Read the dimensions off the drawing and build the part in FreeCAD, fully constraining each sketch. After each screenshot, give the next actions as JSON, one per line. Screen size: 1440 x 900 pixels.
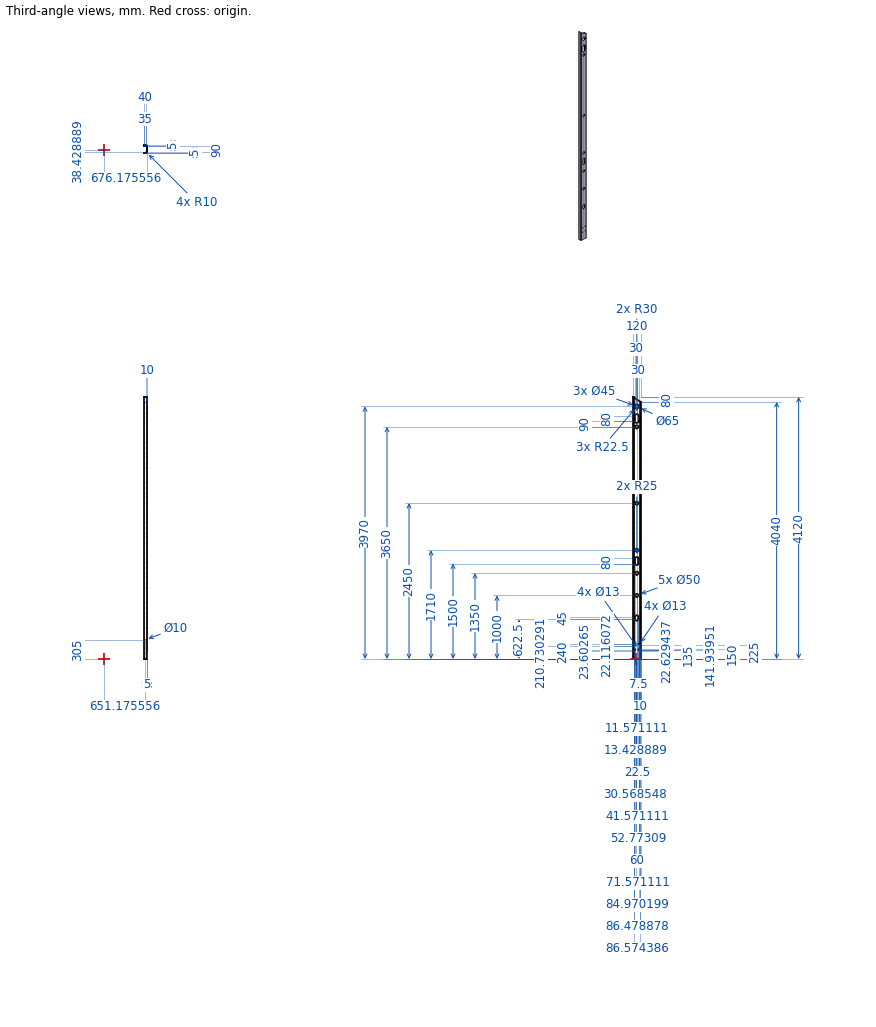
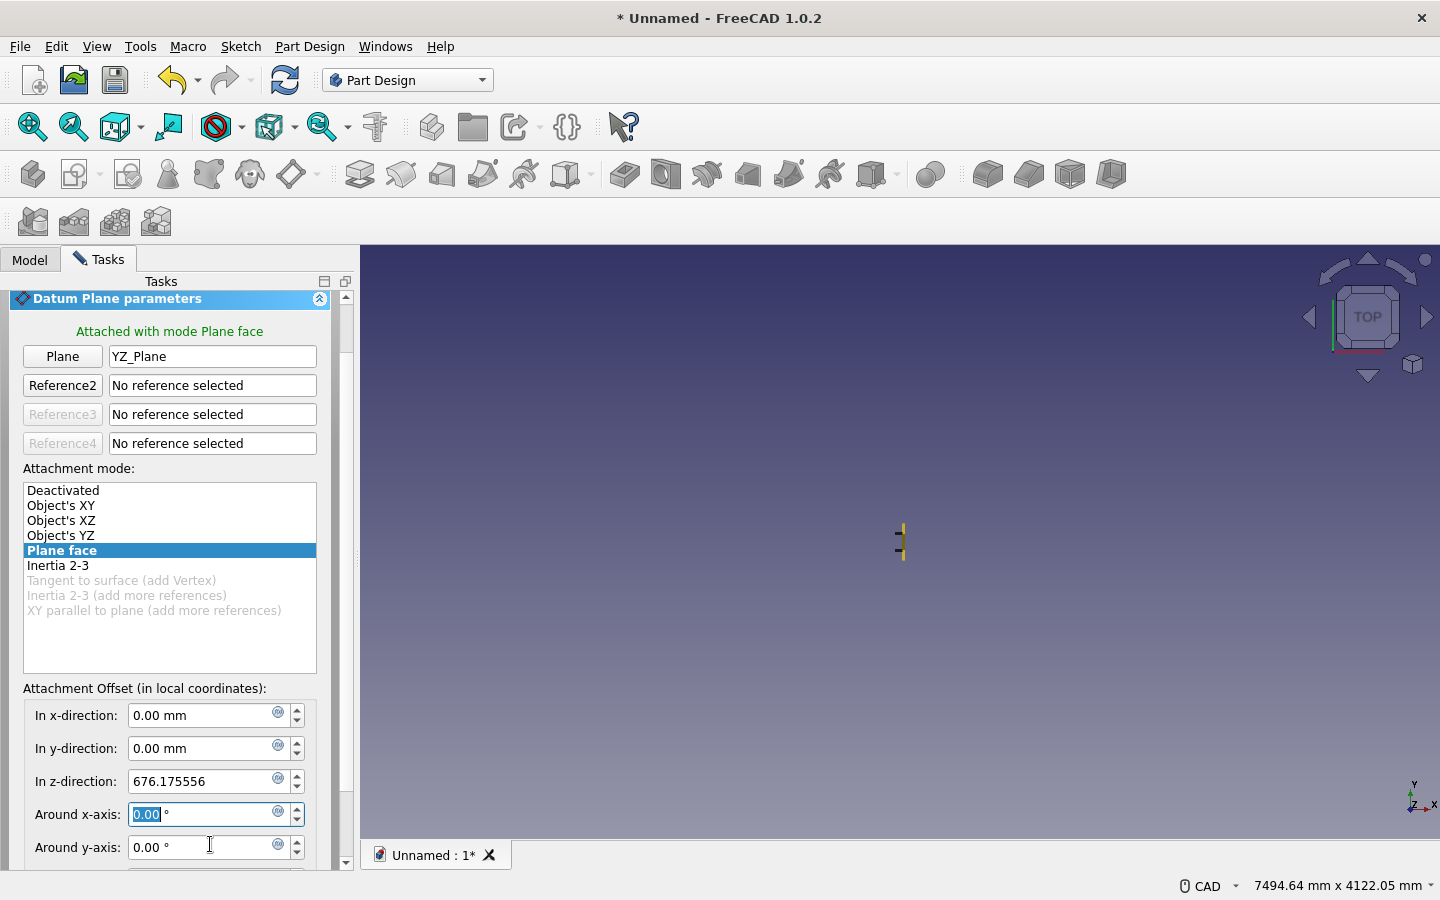
{"action": "scroll", "coordinate": [346, 580], "scroll_direction": "up", "scroll_amount": 2}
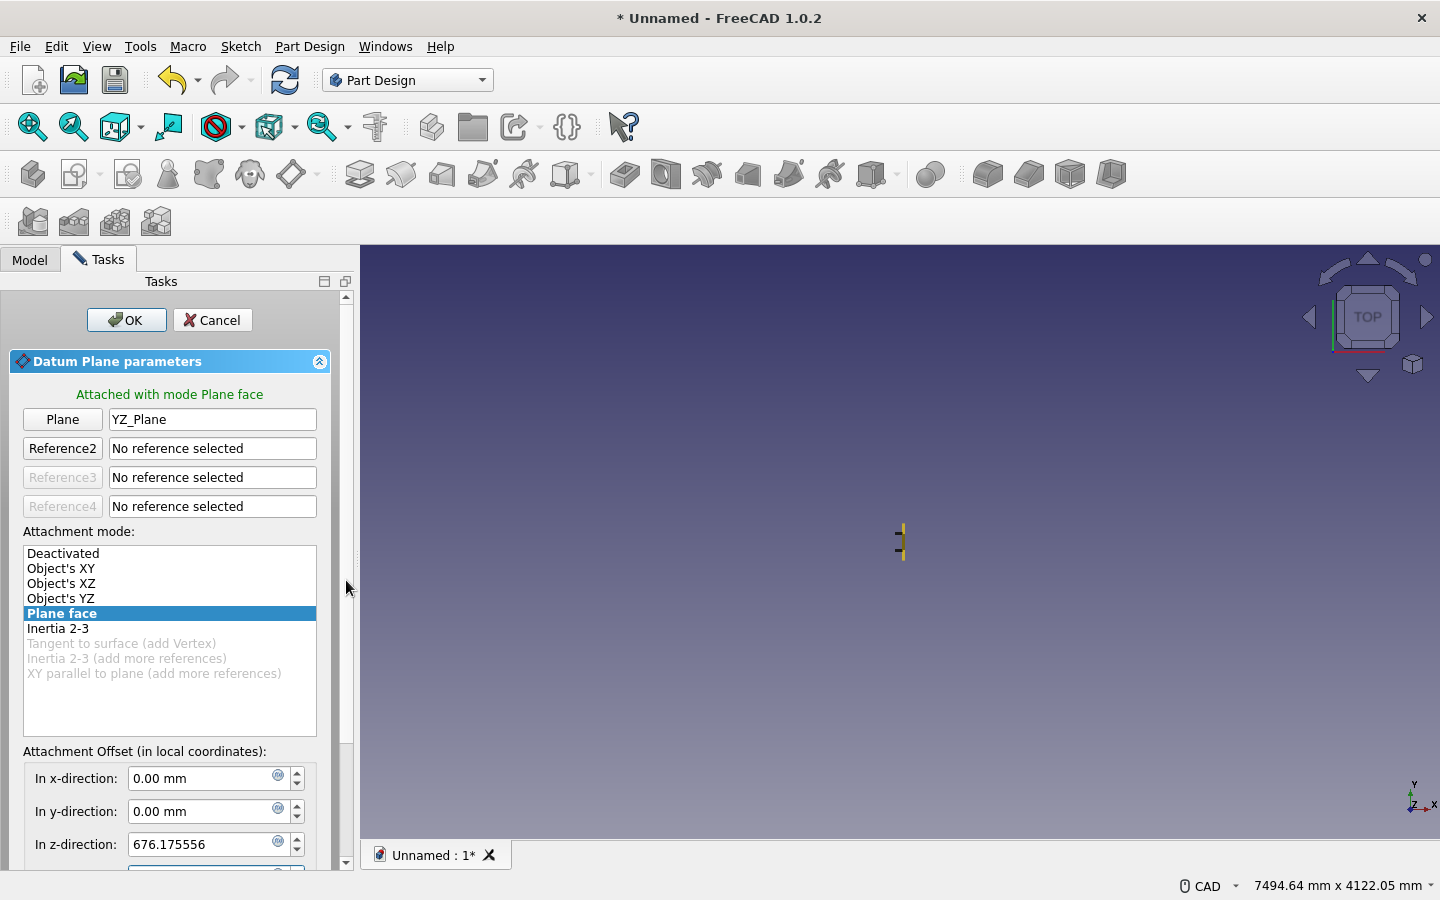
{"action": "left_click", "coordinate": [127, 320]}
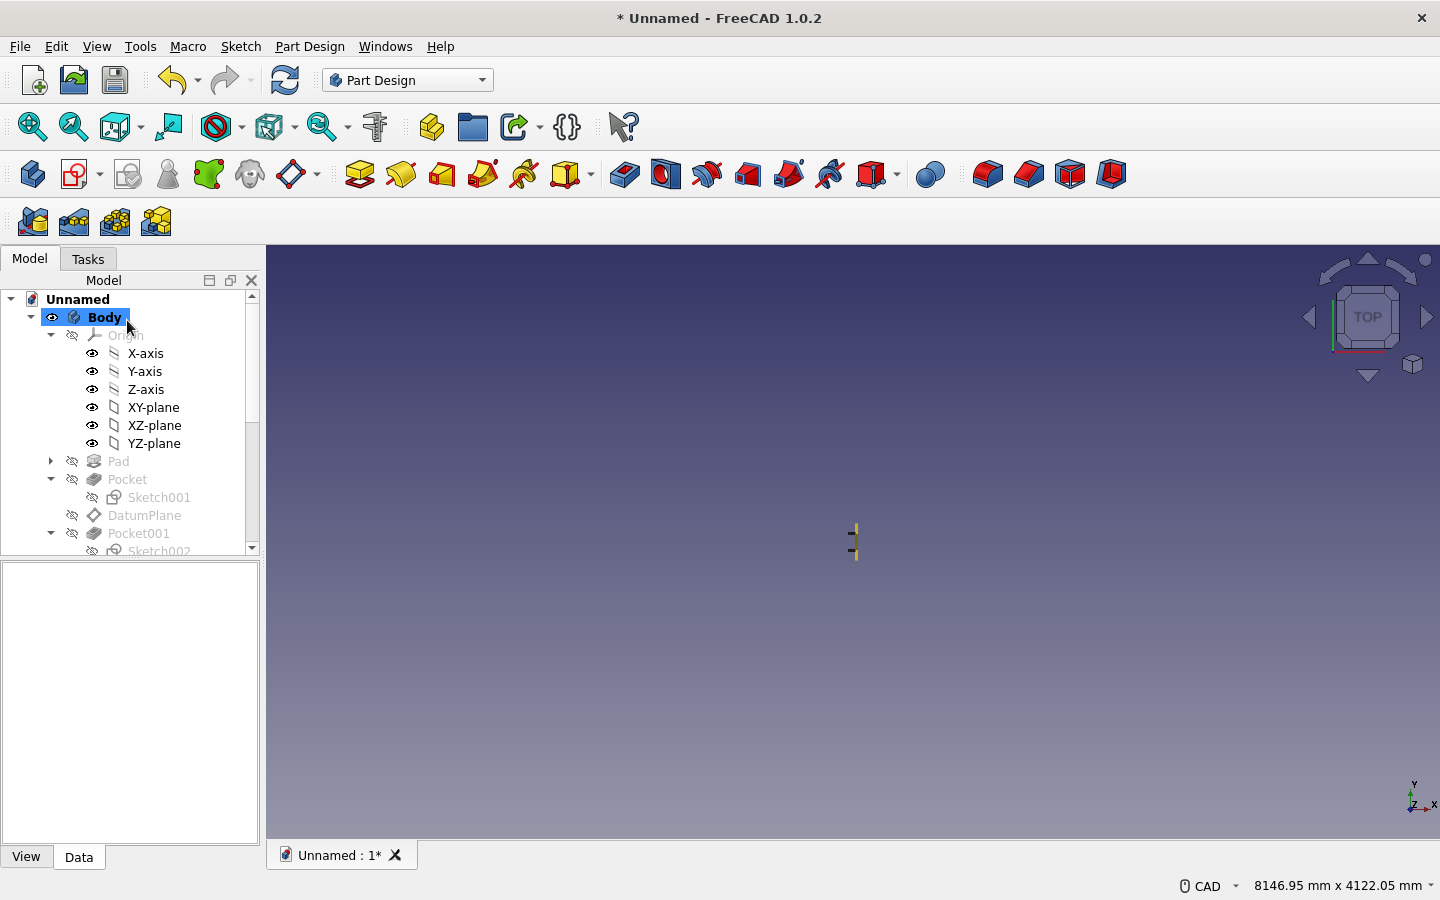
{"action": "scroll", "coordinate": [101, 421], "scroll_direction": "down", "scroll_amount": 3}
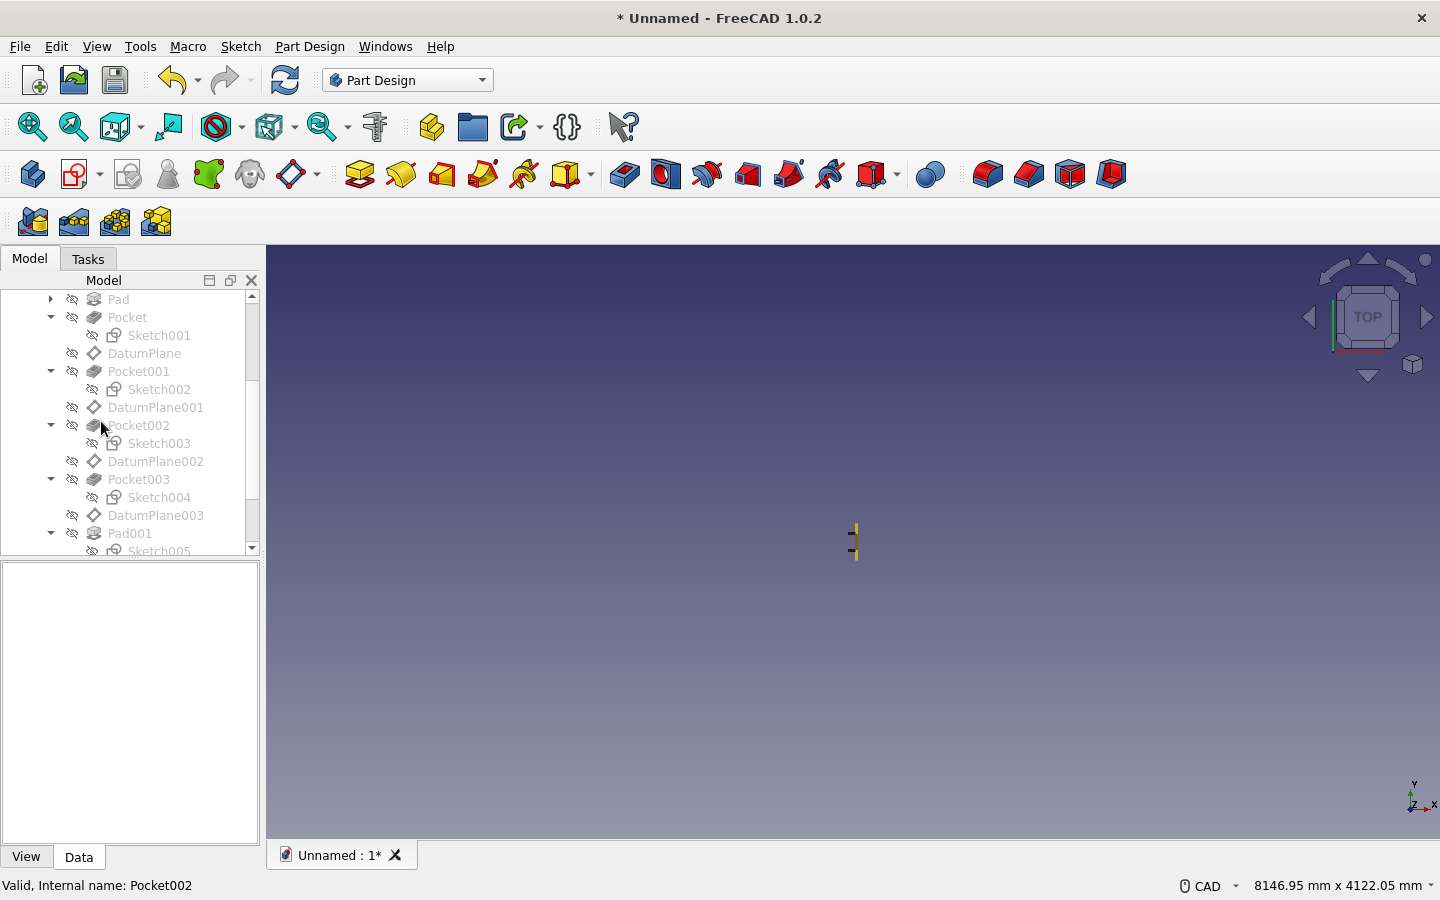
{"action": "scroll", "coordinate": [141, 421], "scroll_direction": "up", "scroll_amount": 15}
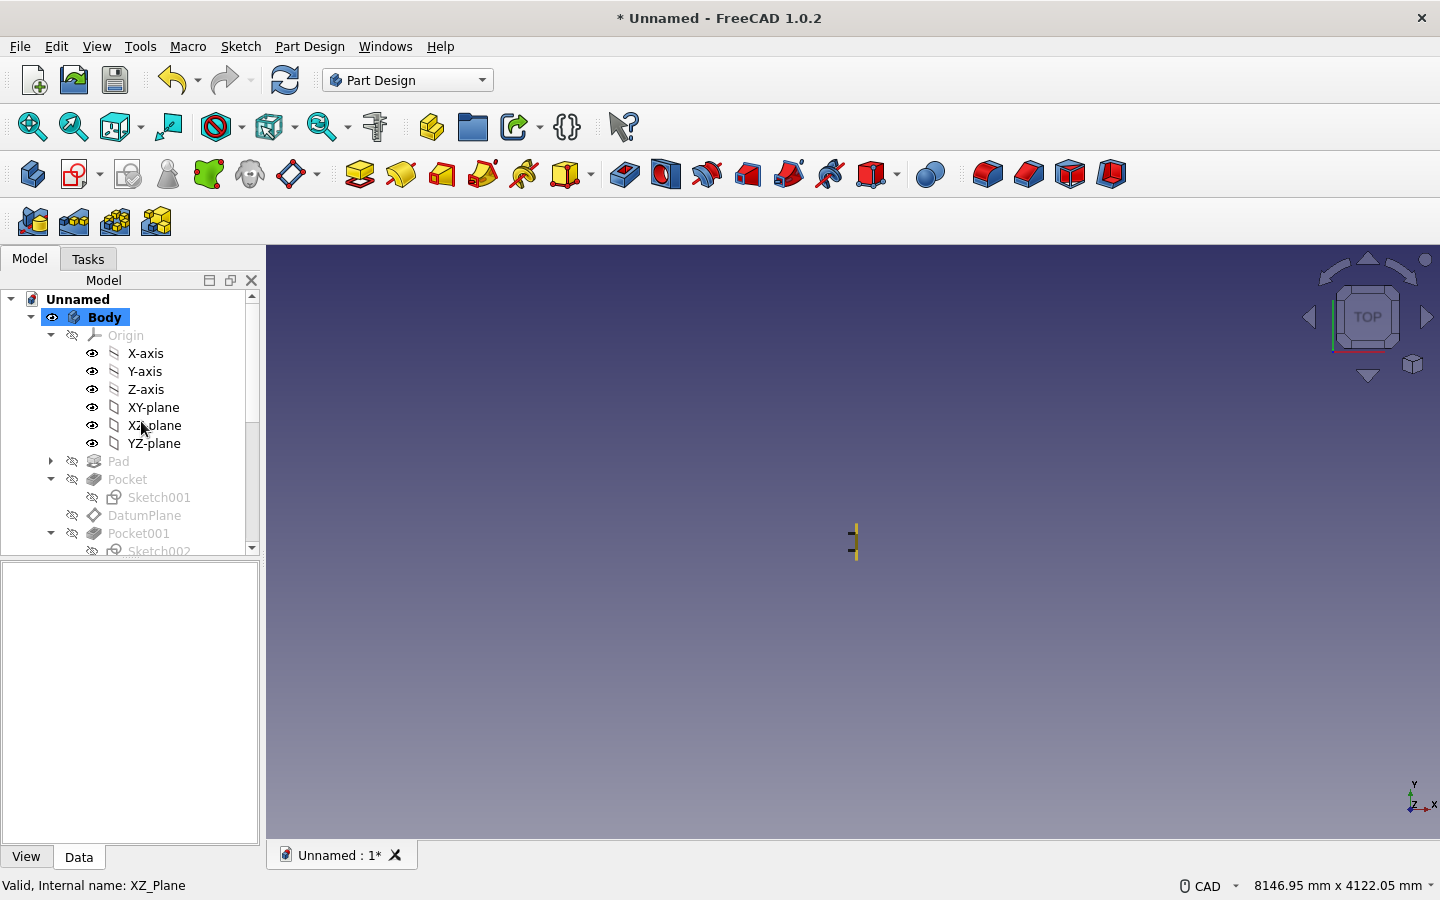
{"action": "scroll", "coordinate": [101, 421], "scroll_direction": "down", "scroll_amount": 6}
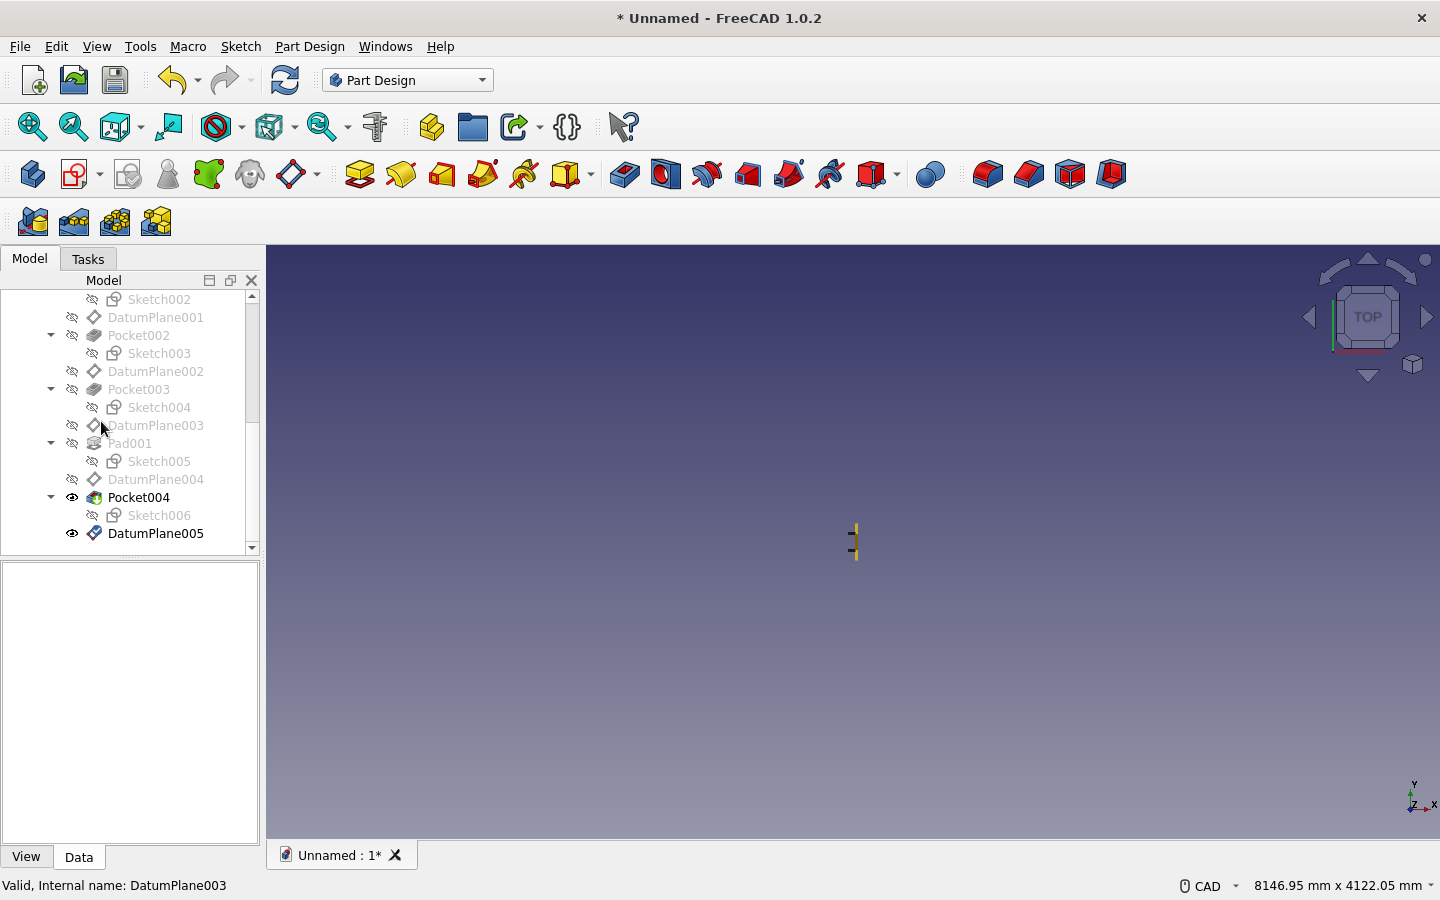
{"action": "left_click", "coordinate": [117, 533]}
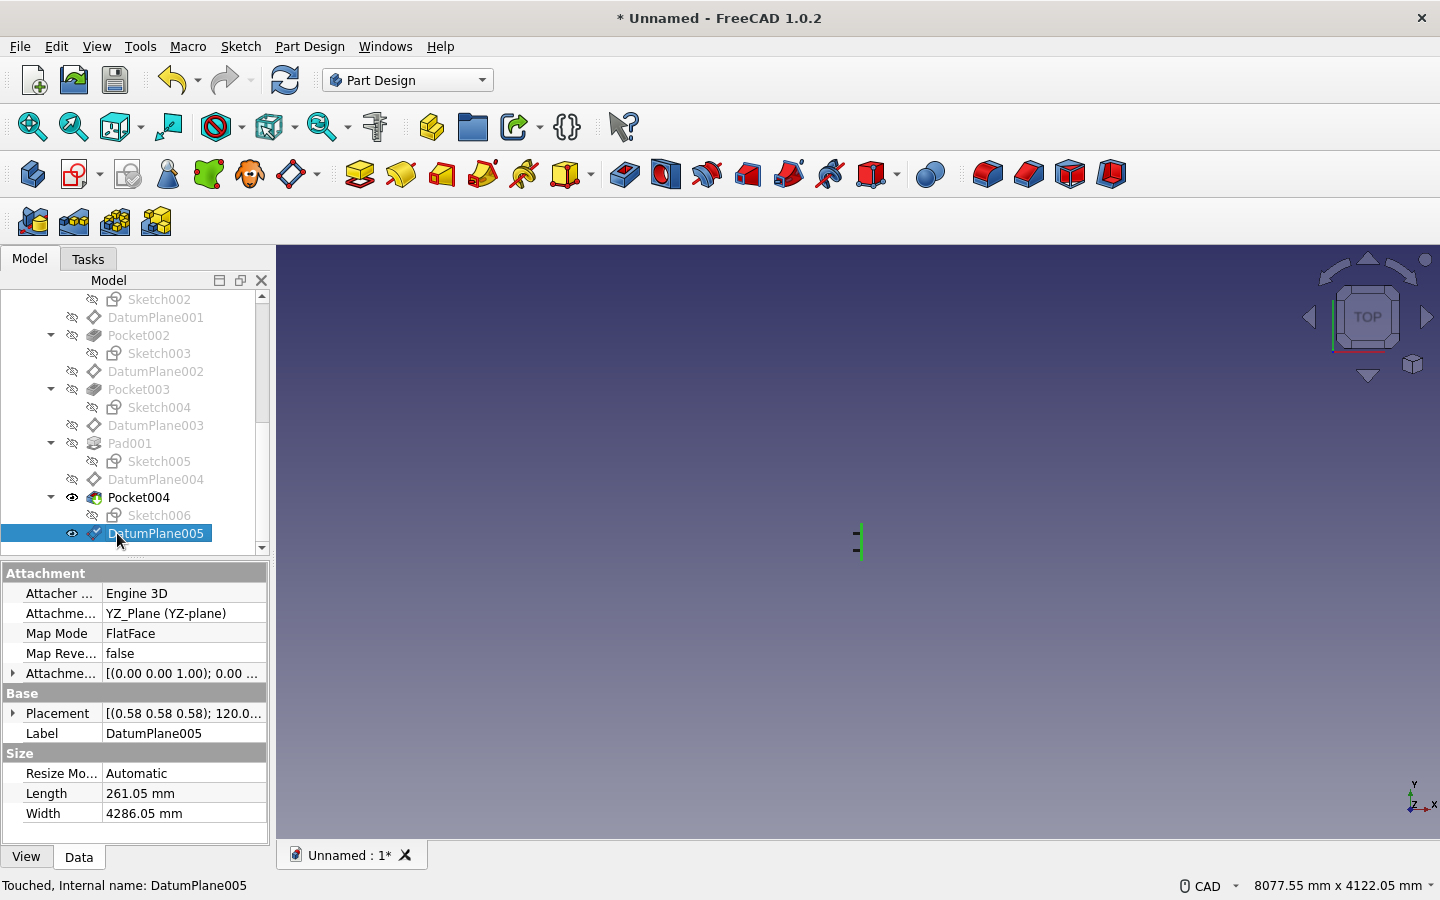
{"action": "left_click", "coordinate": [74, 174]}